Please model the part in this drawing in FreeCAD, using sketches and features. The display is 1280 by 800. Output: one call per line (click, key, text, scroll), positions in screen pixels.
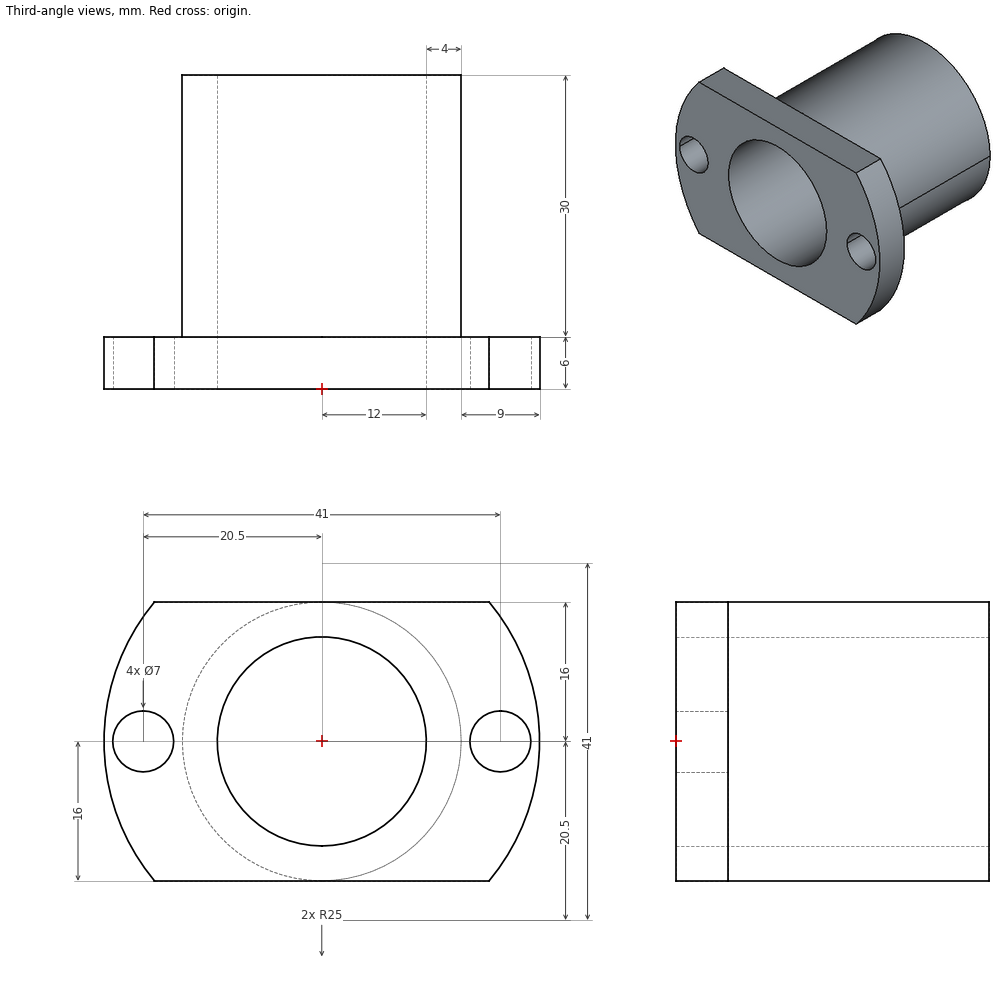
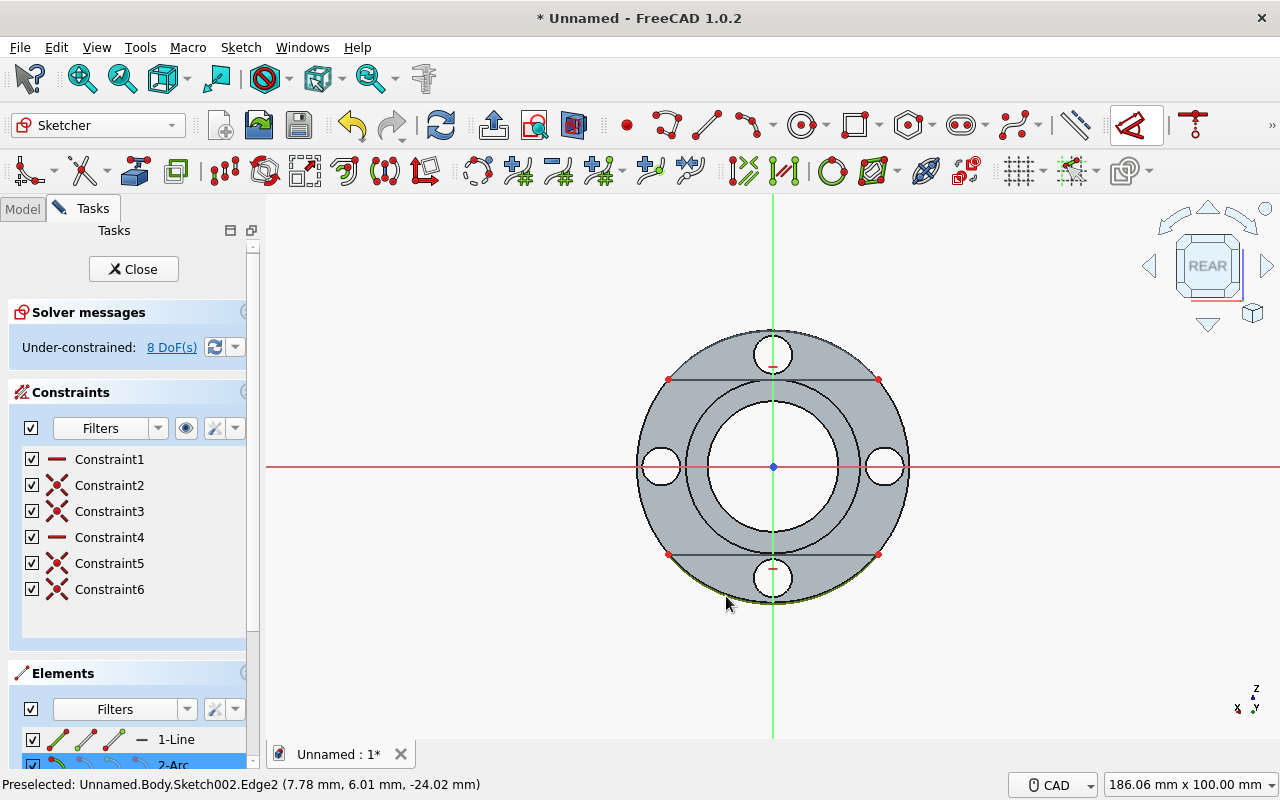
click(820, 339)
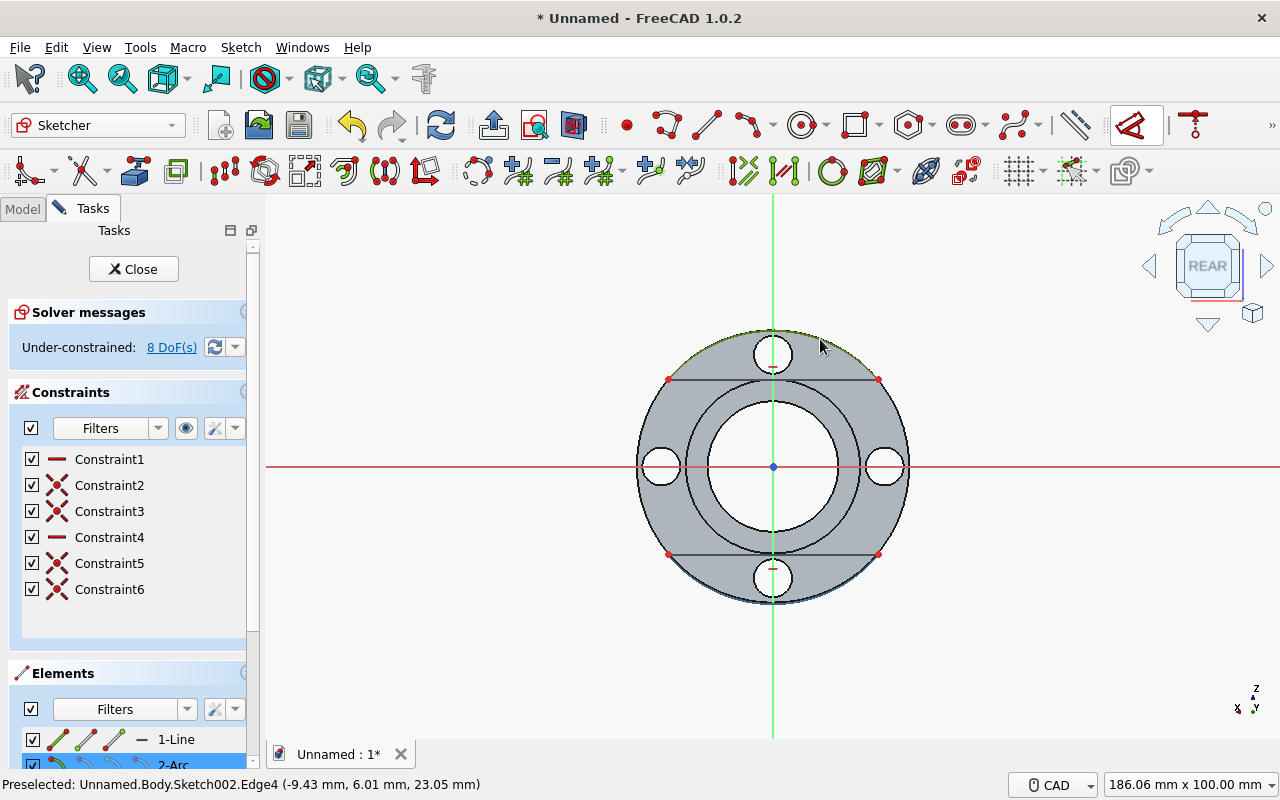
click(1194, 126)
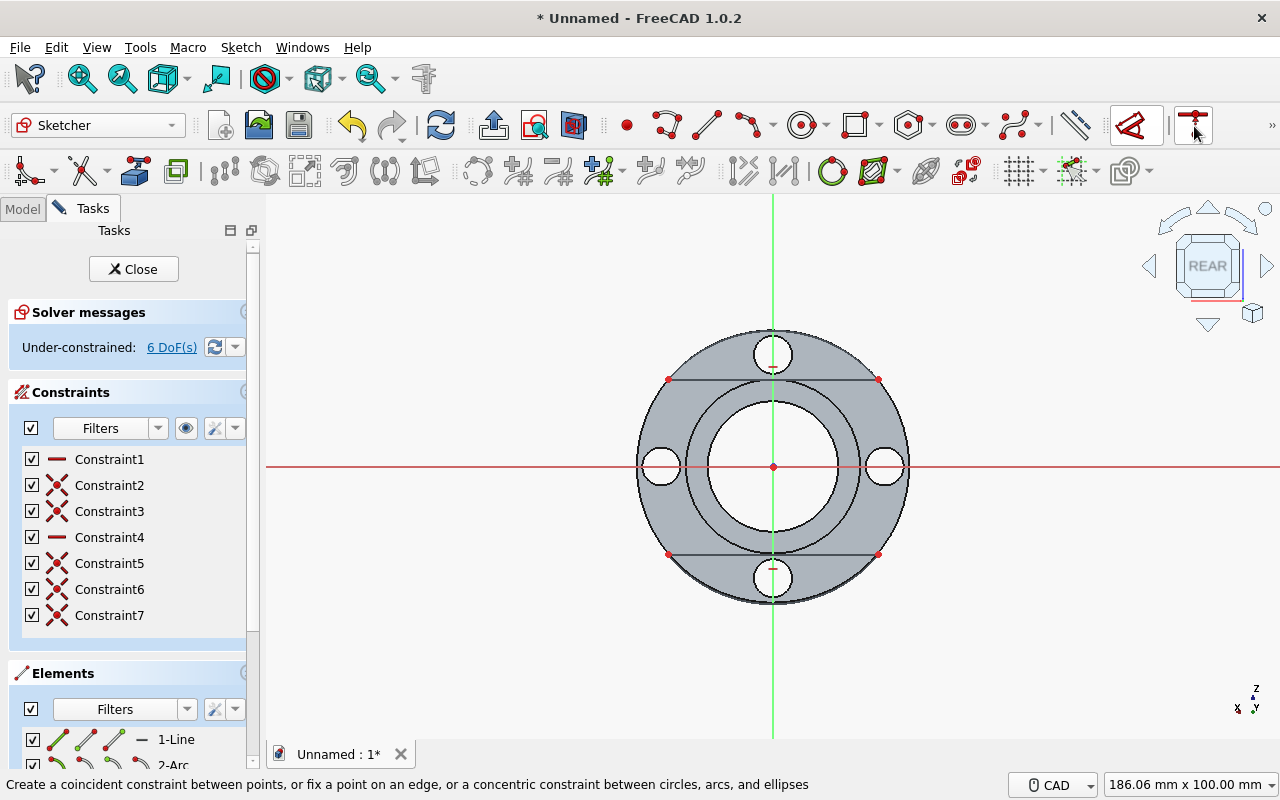
drag(763, 457, 783, 478)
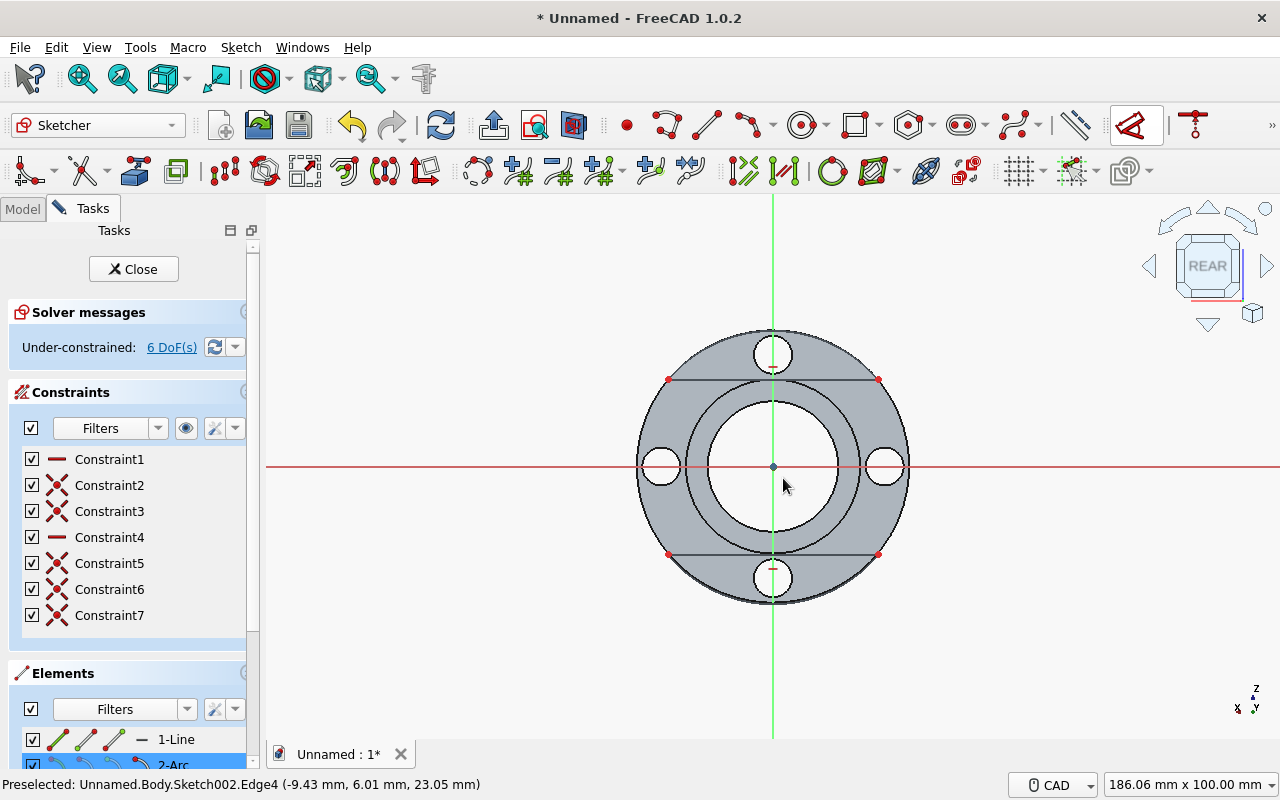
click(1194, 126)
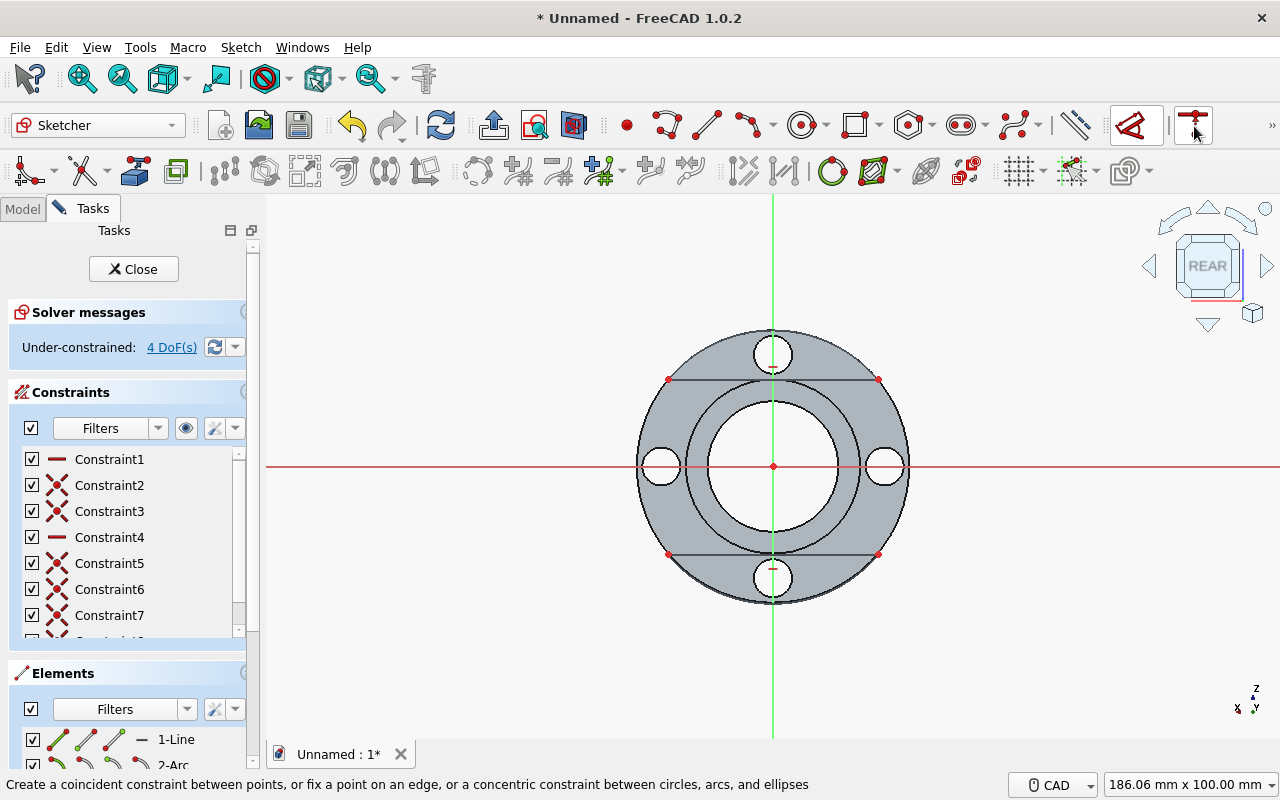
click(726, 596)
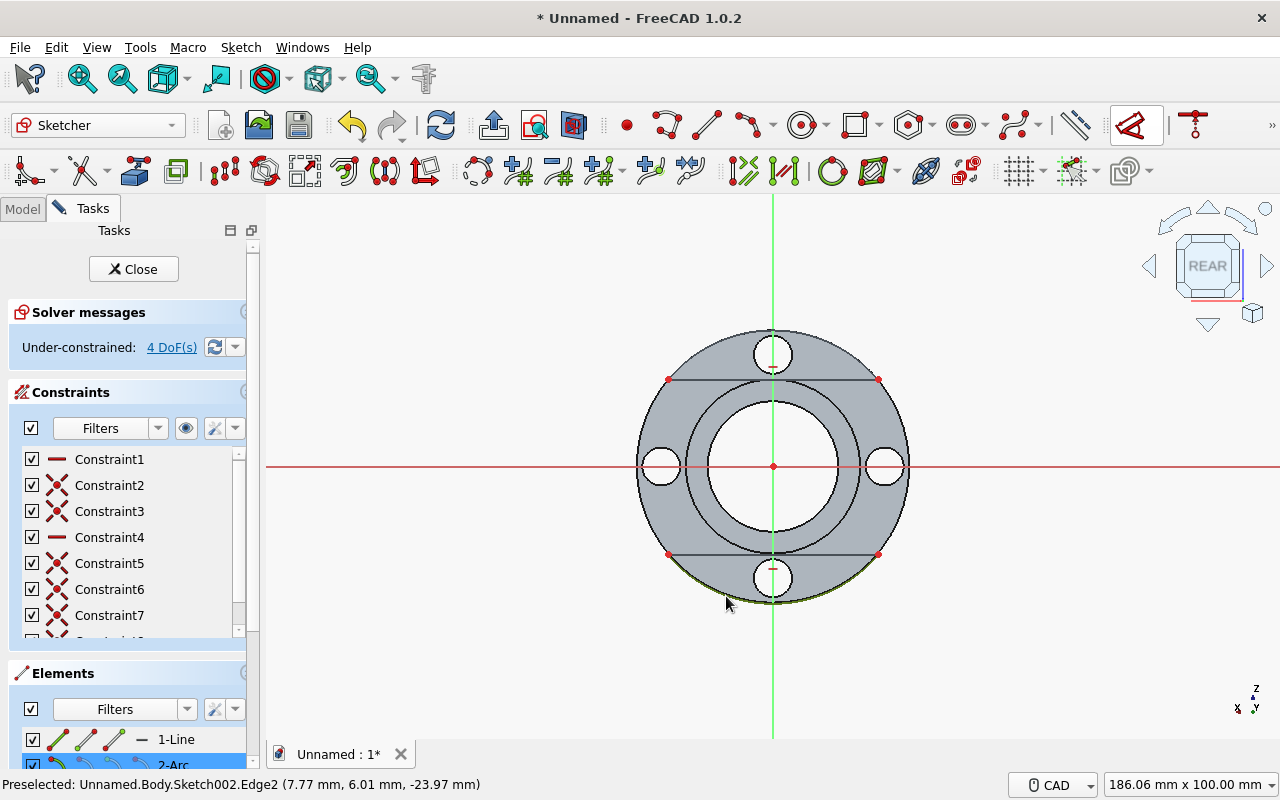
click(820, 339)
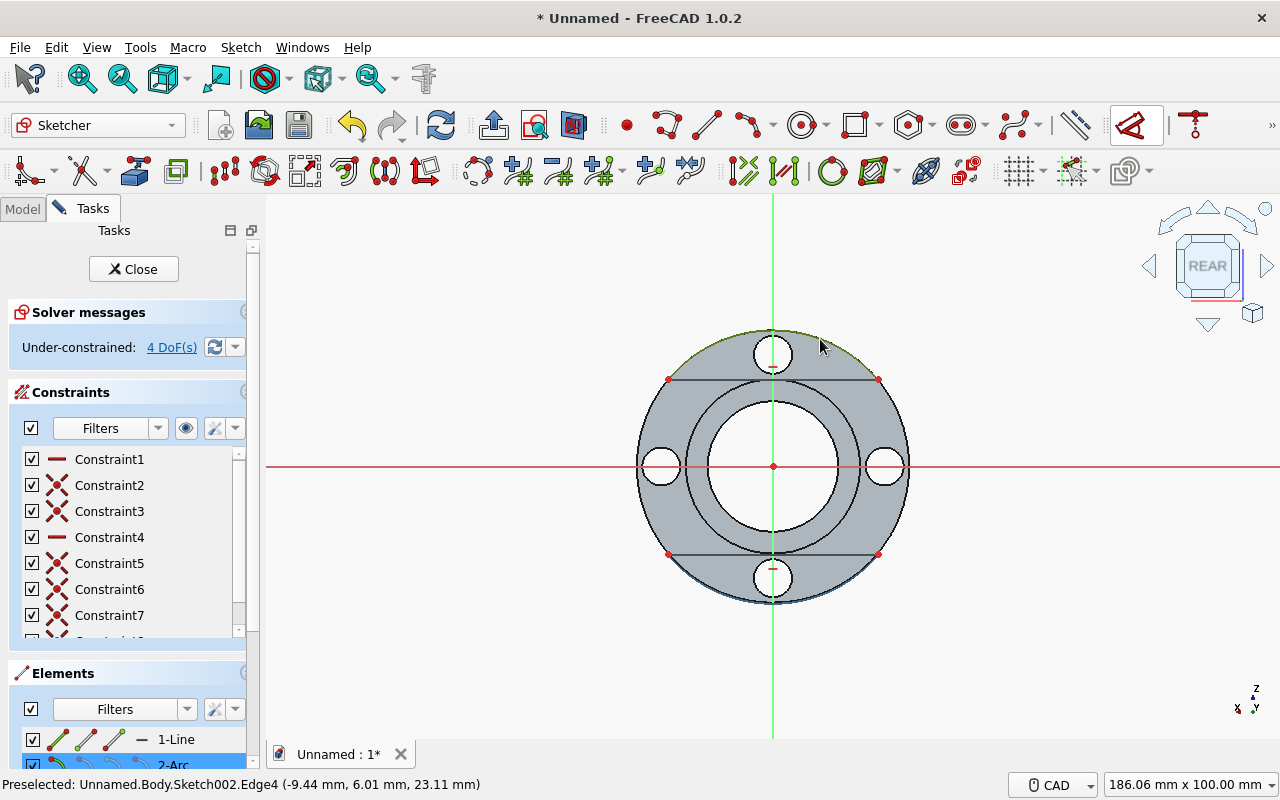
key(e)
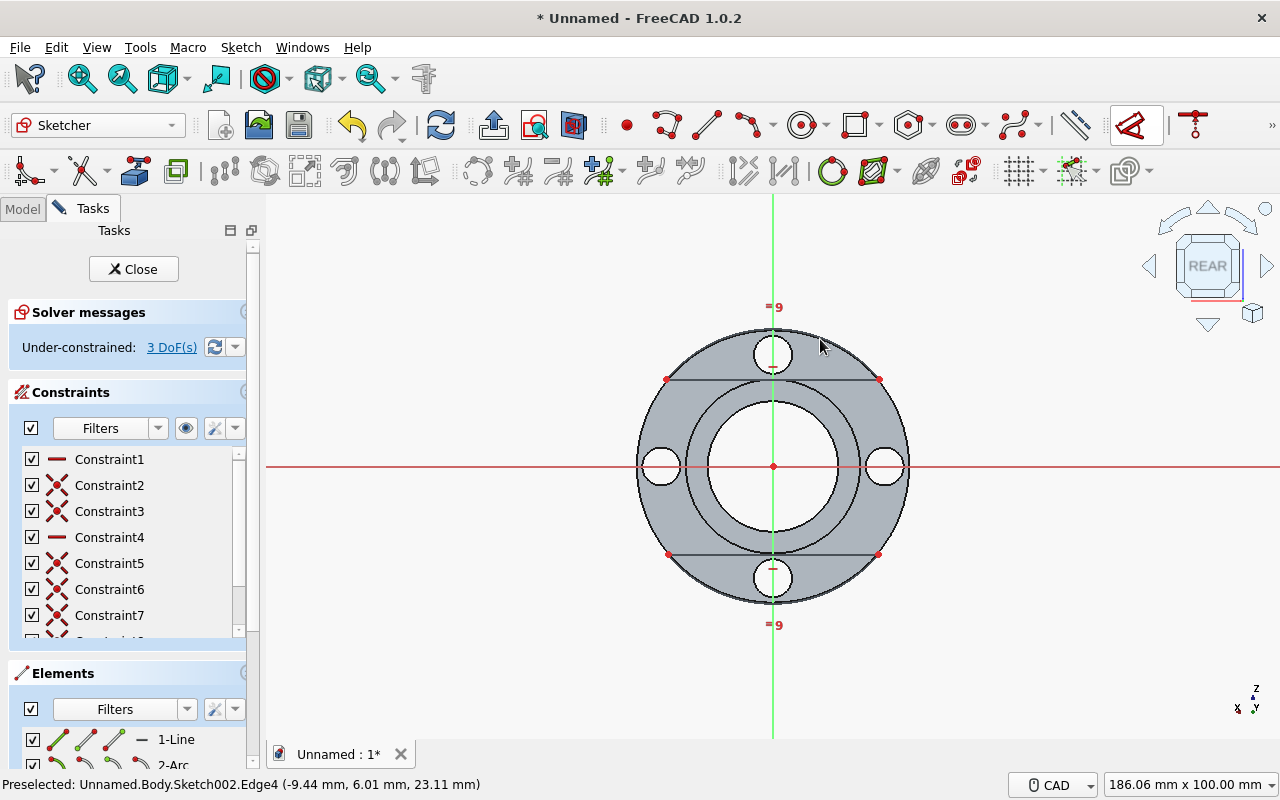
click(726, 596)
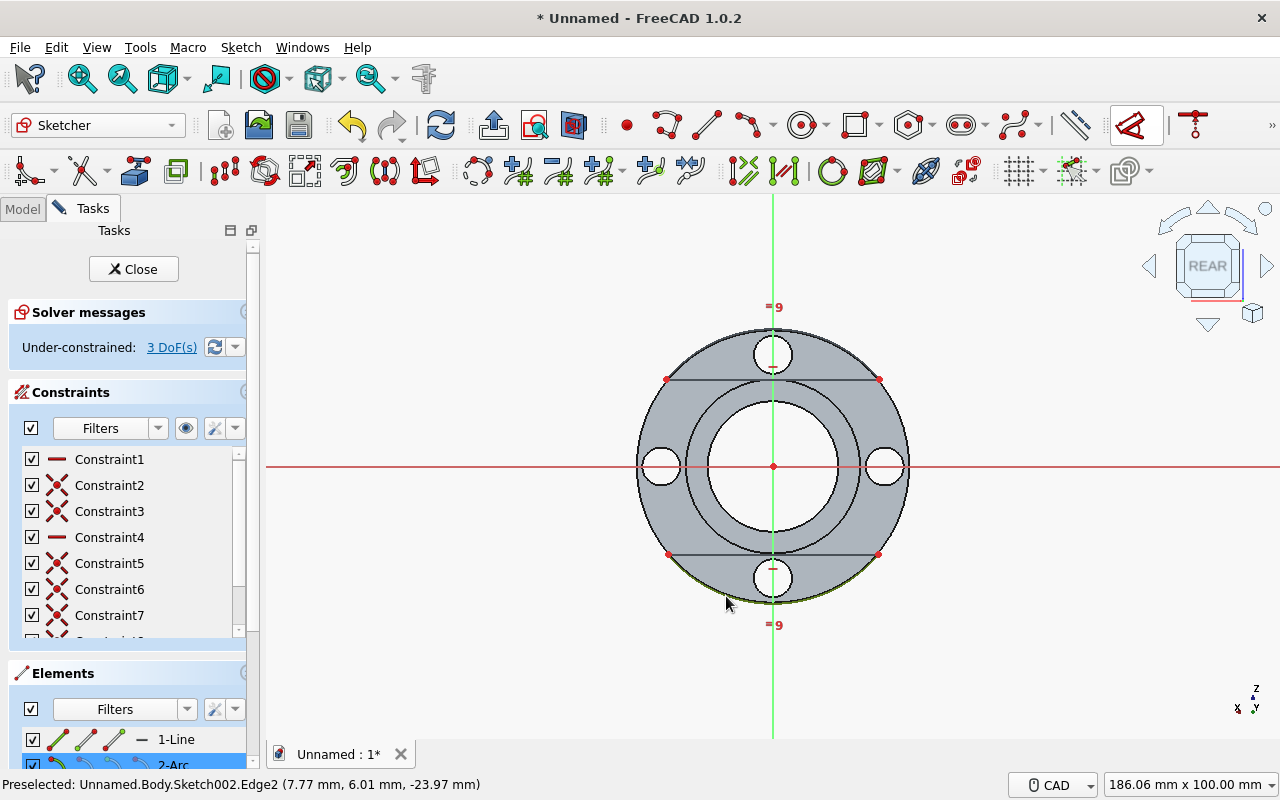
click(1158, 126)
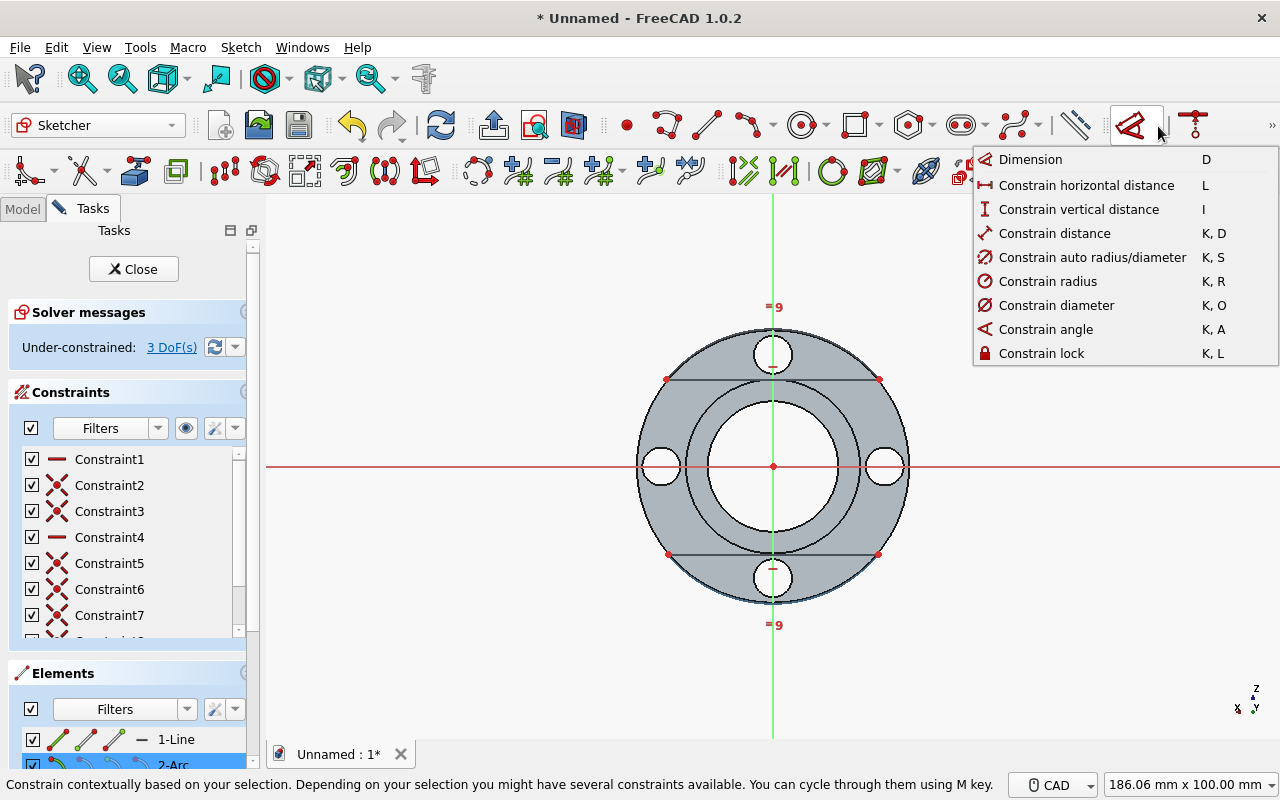
click(1126, 281)